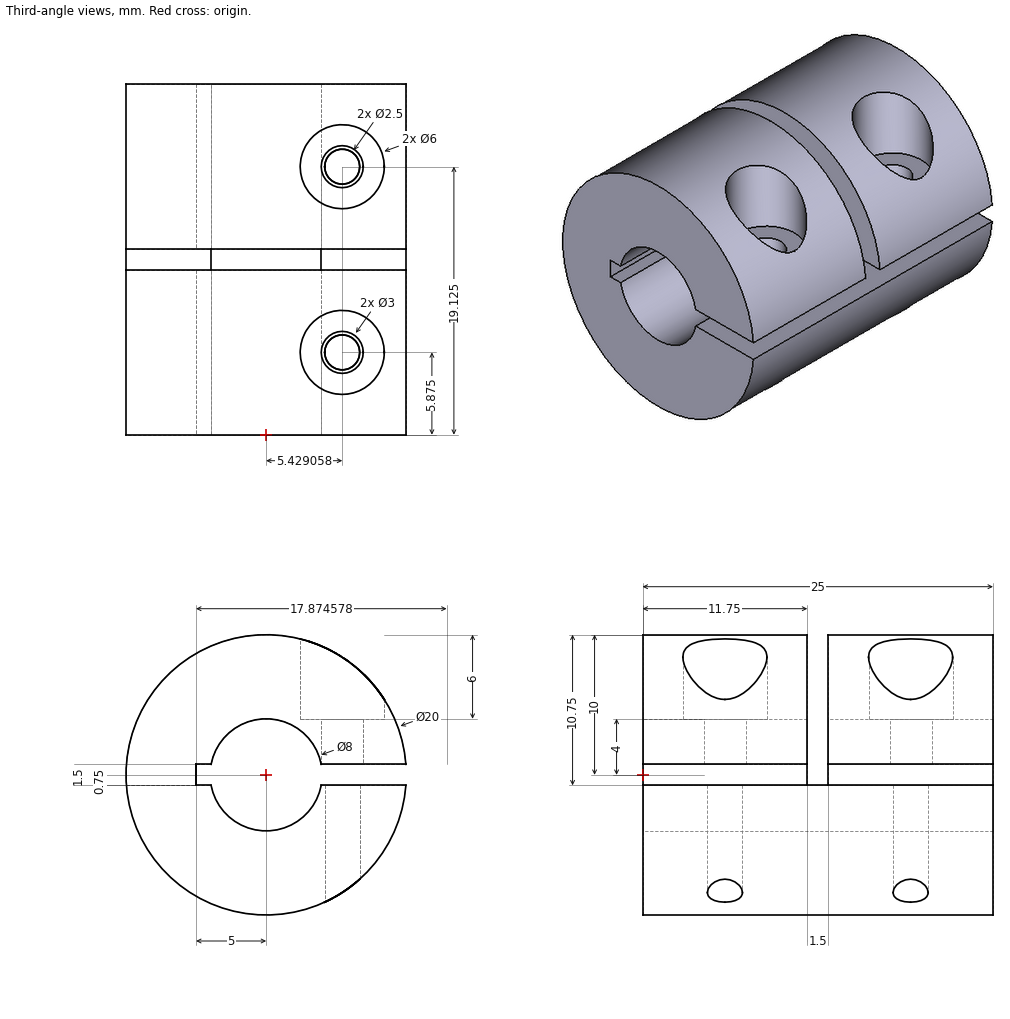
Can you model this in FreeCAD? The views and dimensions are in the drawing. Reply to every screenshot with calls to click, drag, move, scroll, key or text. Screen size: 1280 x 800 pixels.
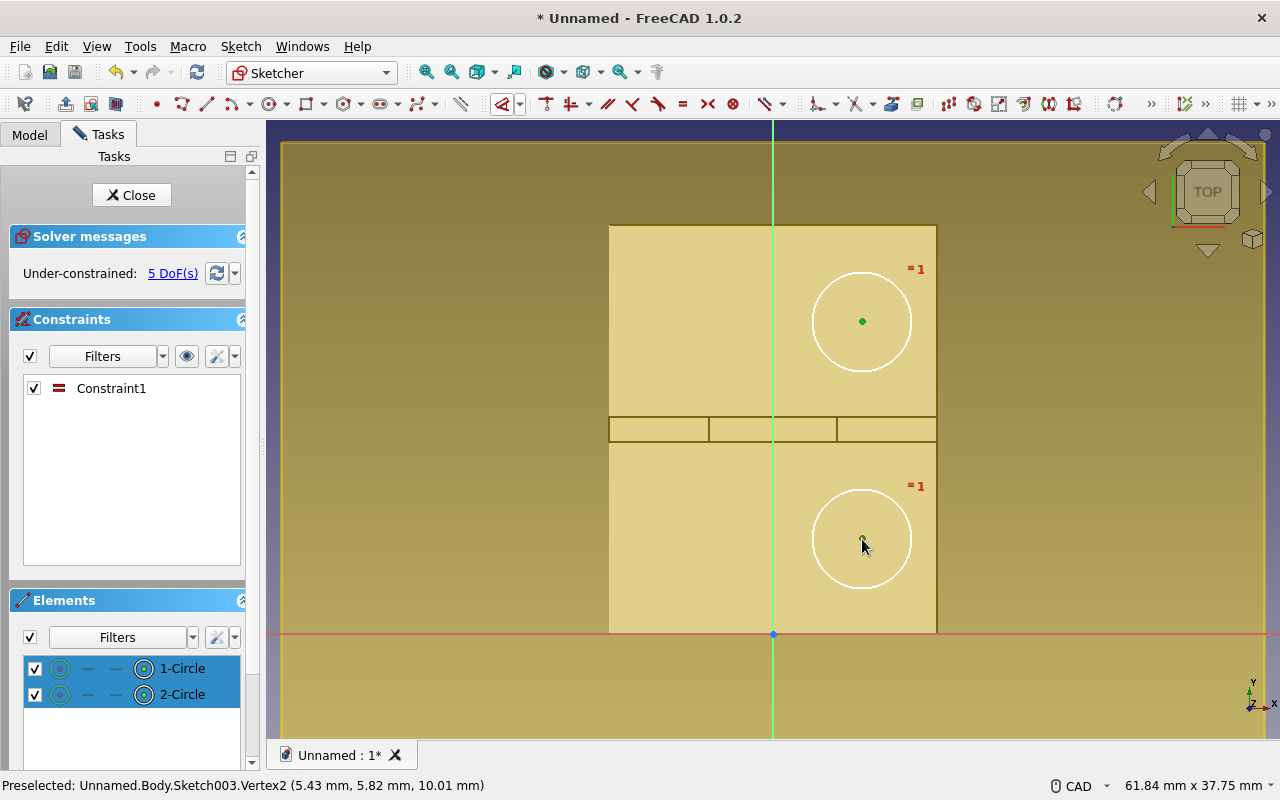
click(588, 104)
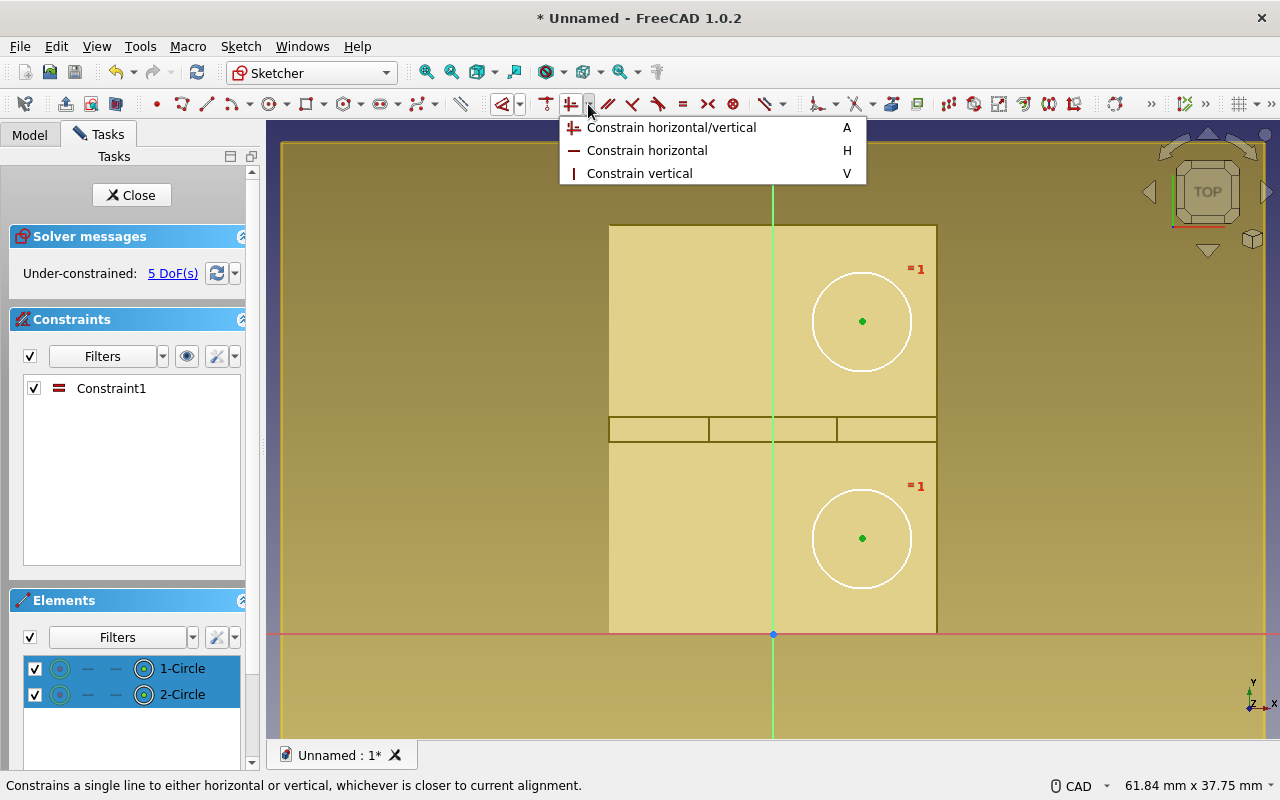
click(713, 174)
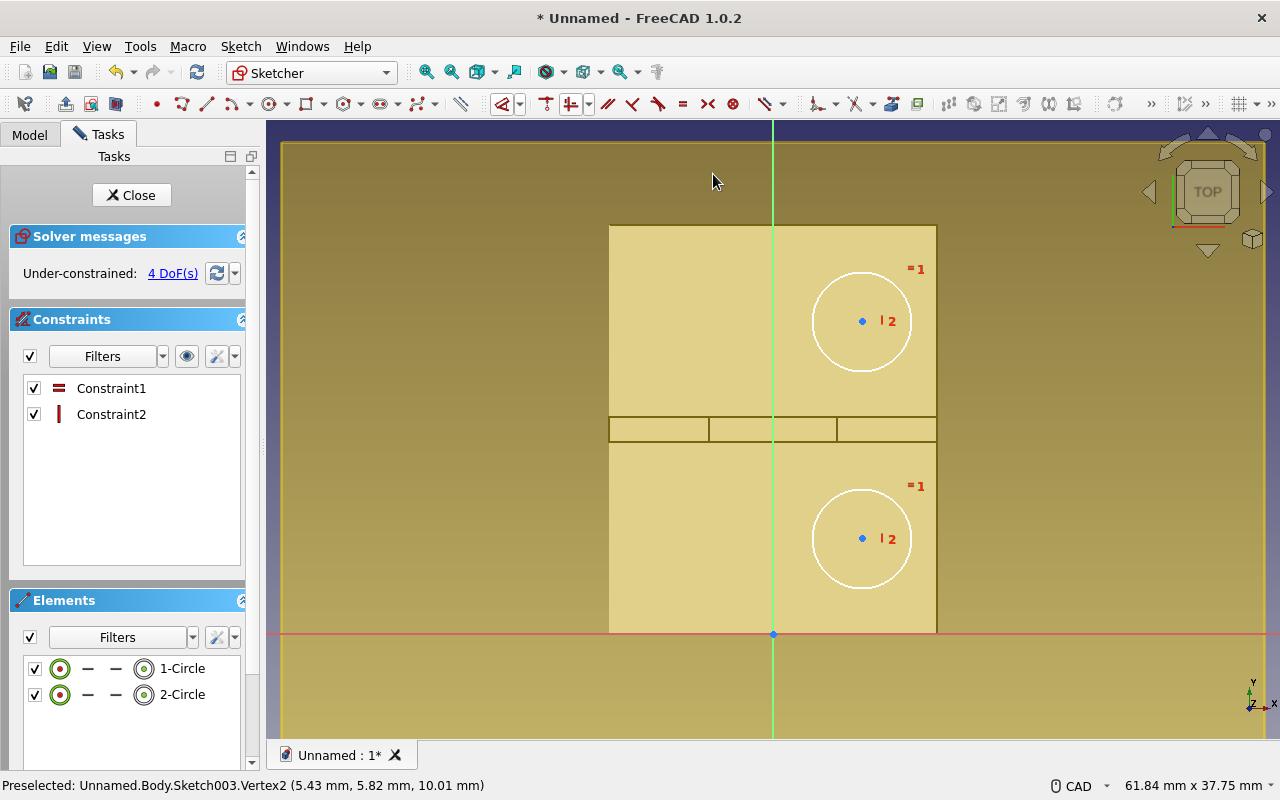
click(897, 287)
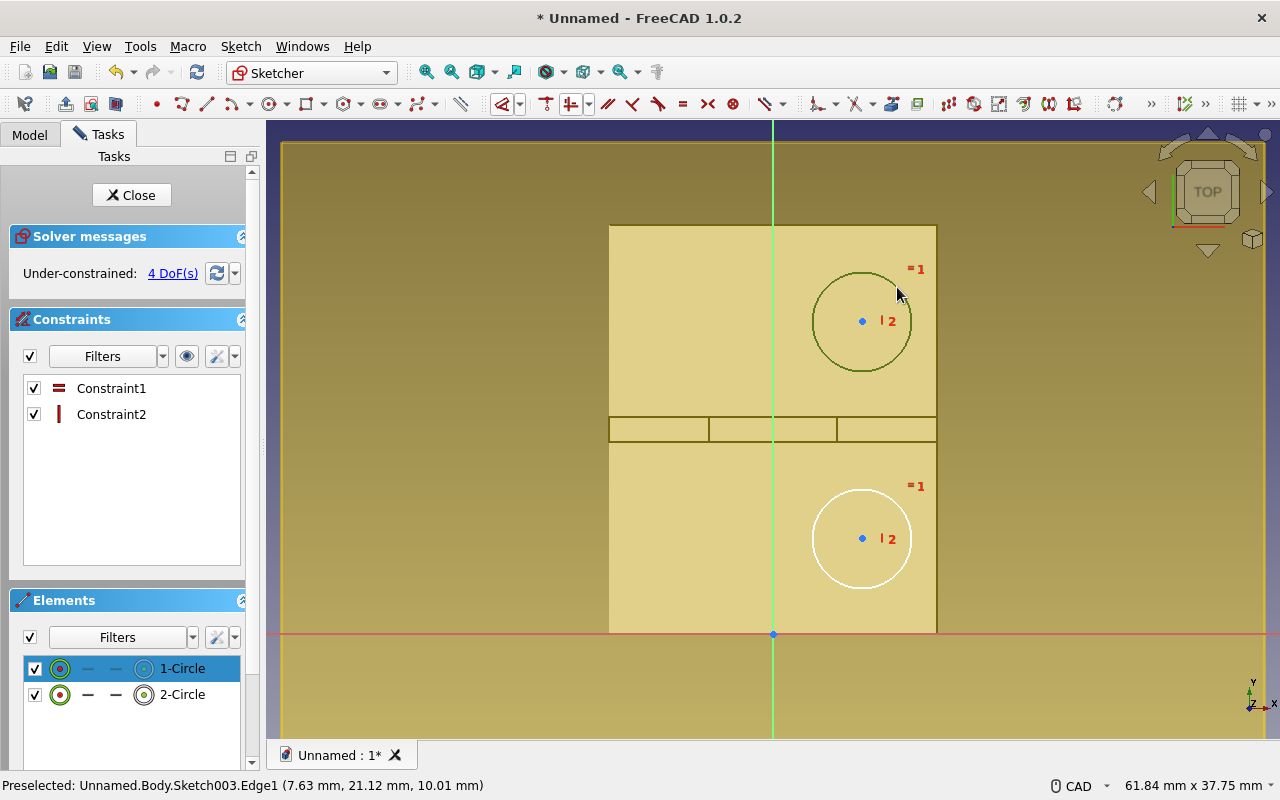
click(520, 104)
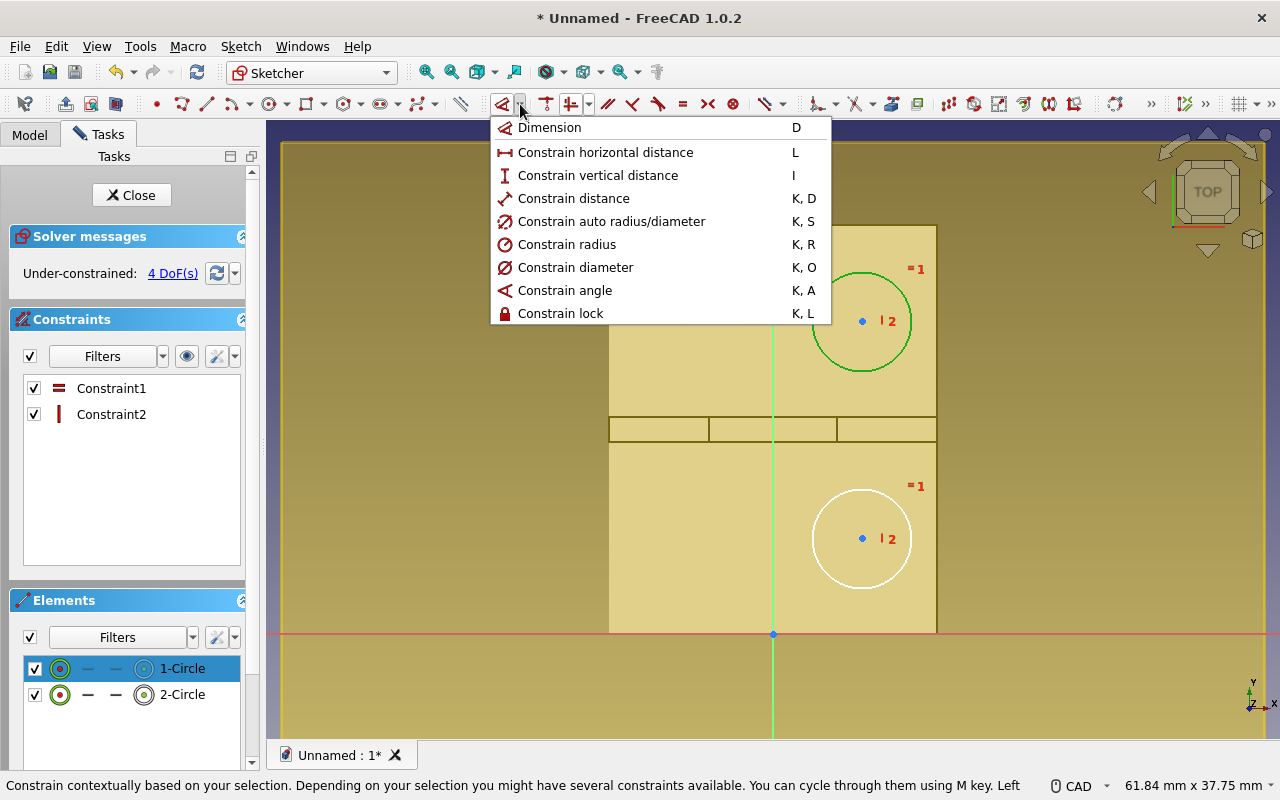
click(661, 268)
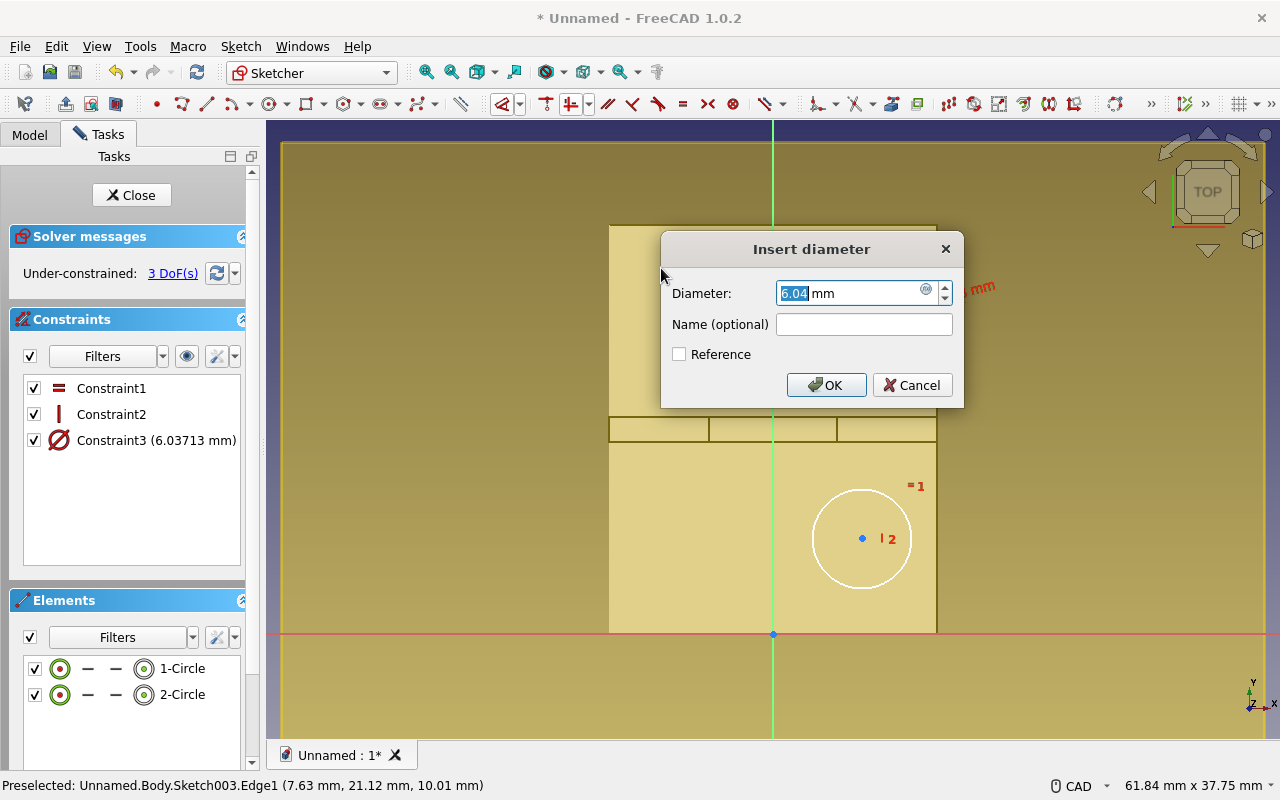
text(6)
key(Return)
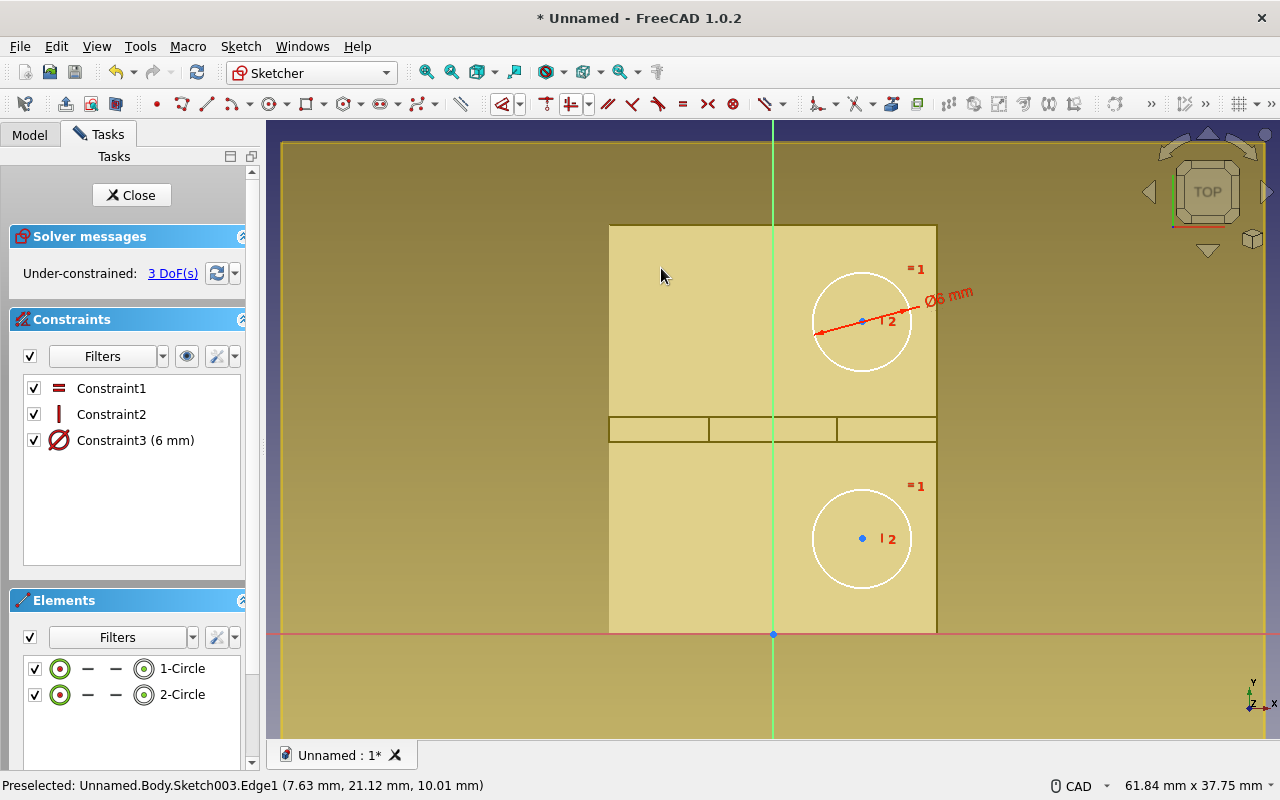
click(862, 539)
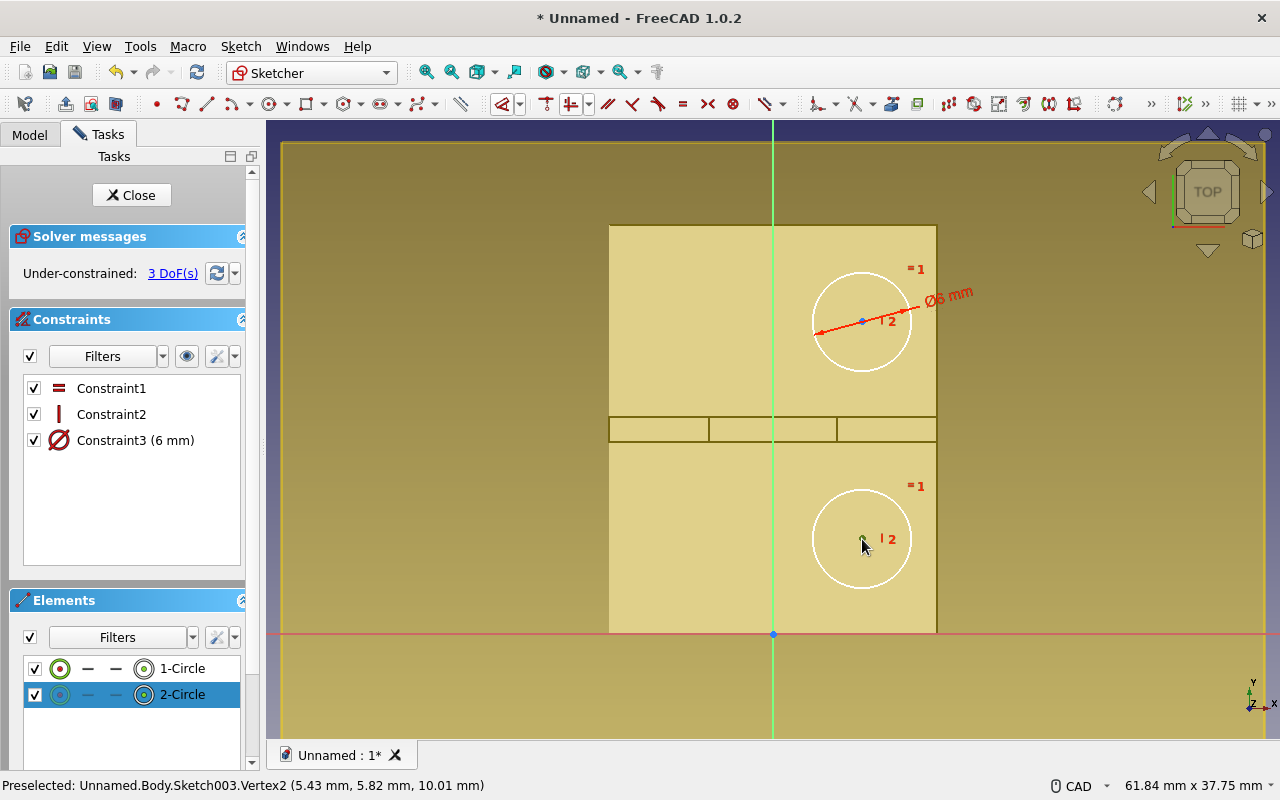
click(520, 104)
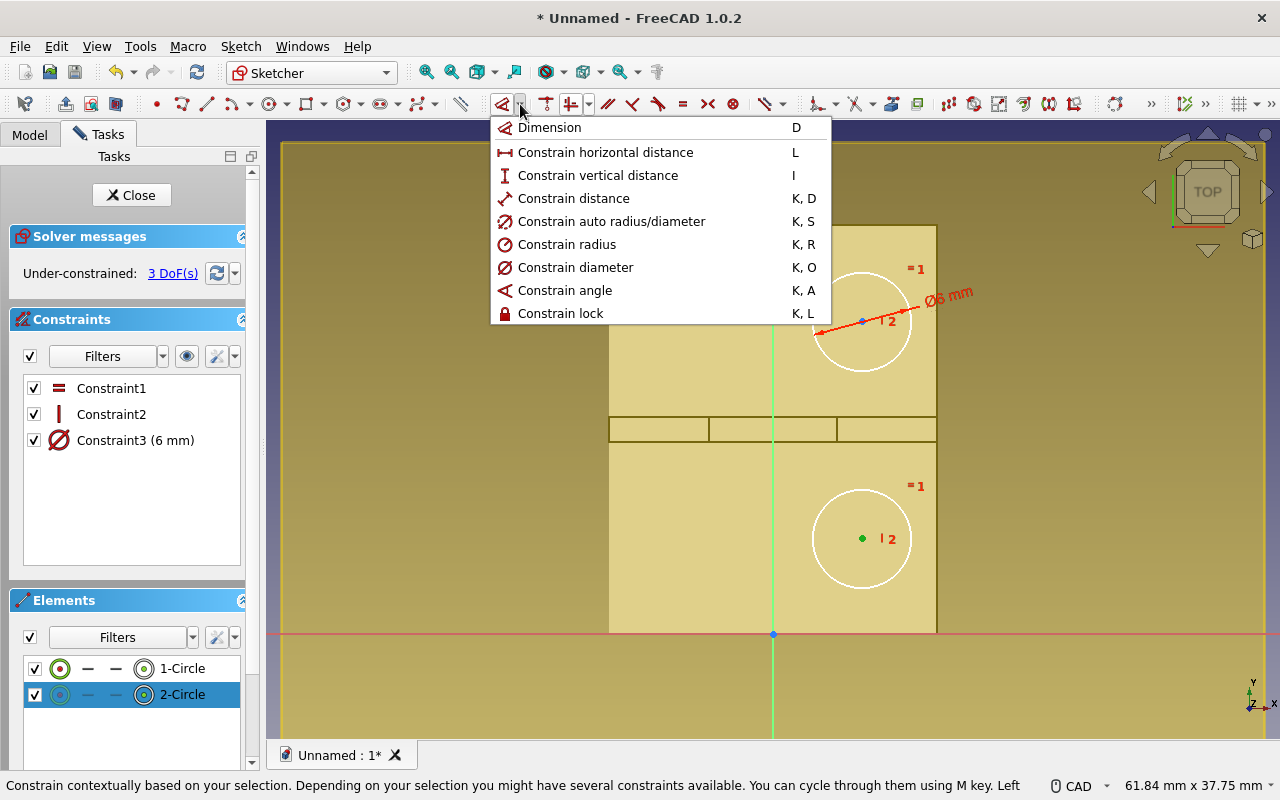
click(661, 176)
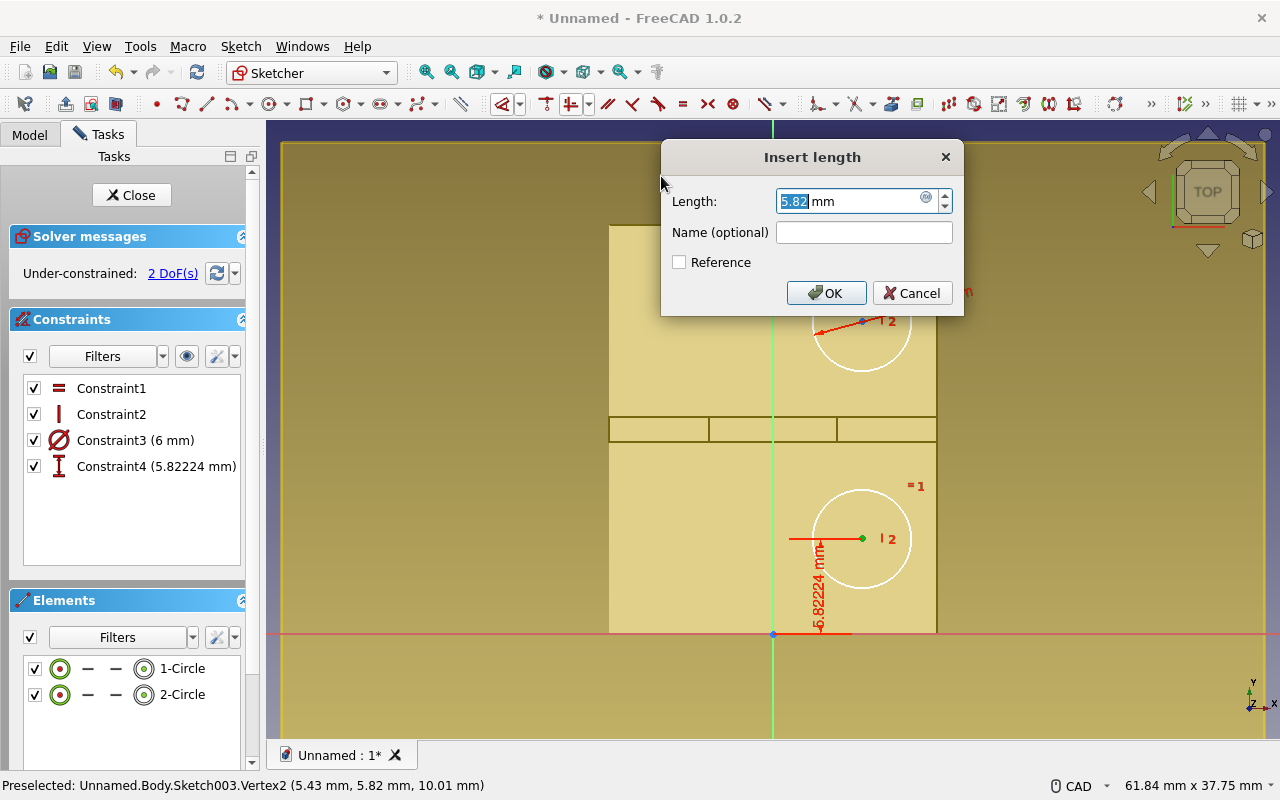
text(5.875)
key(Return)